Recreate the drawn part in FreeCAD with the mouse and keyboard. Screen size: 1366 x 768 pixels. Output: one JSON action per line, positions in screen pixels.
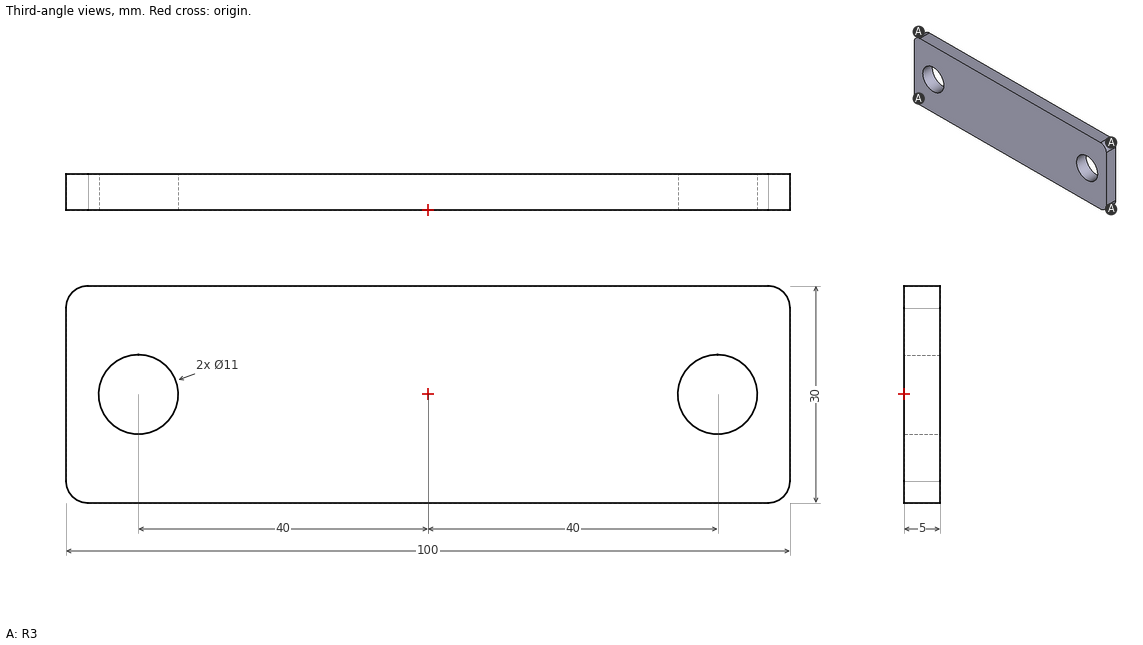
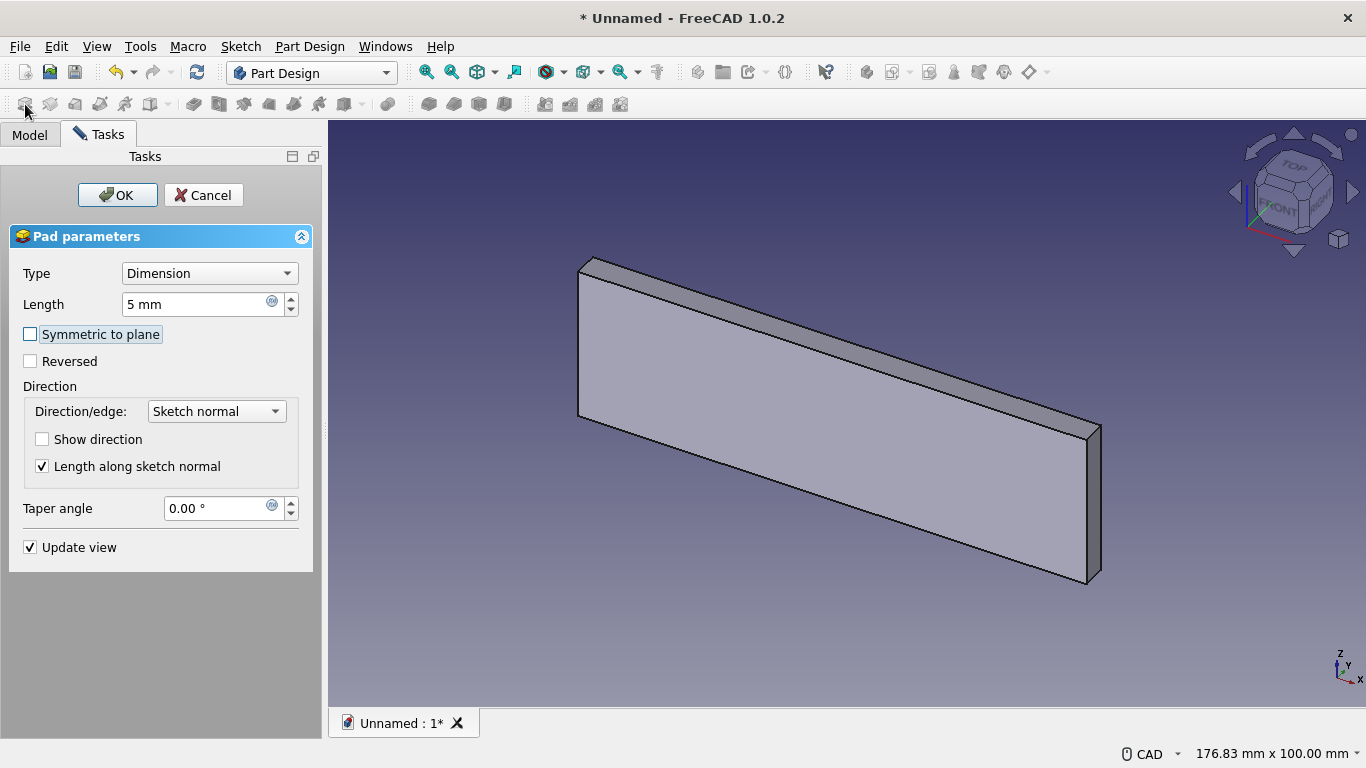
{"action": "left_click", "coordinate": [31, 361]}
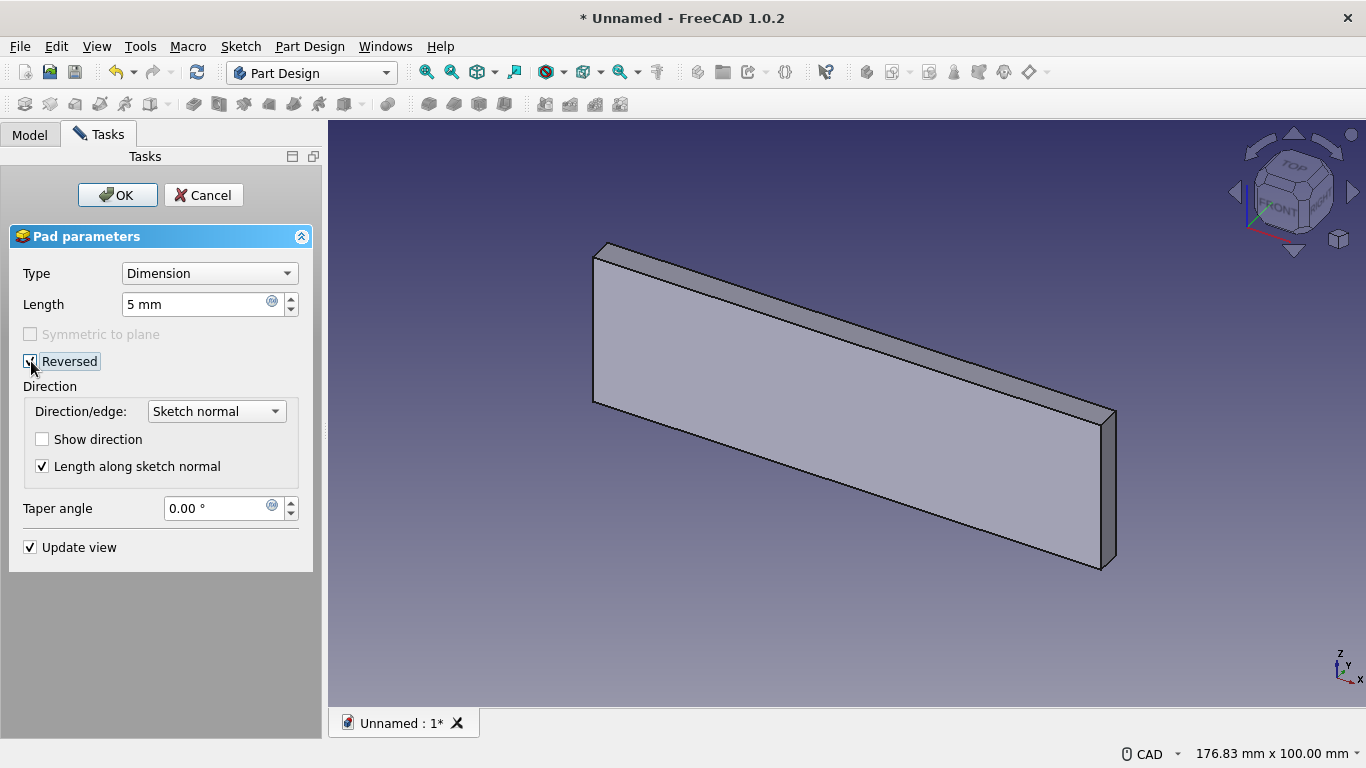
{"action": "left_click", "coordinate": [118, 195]}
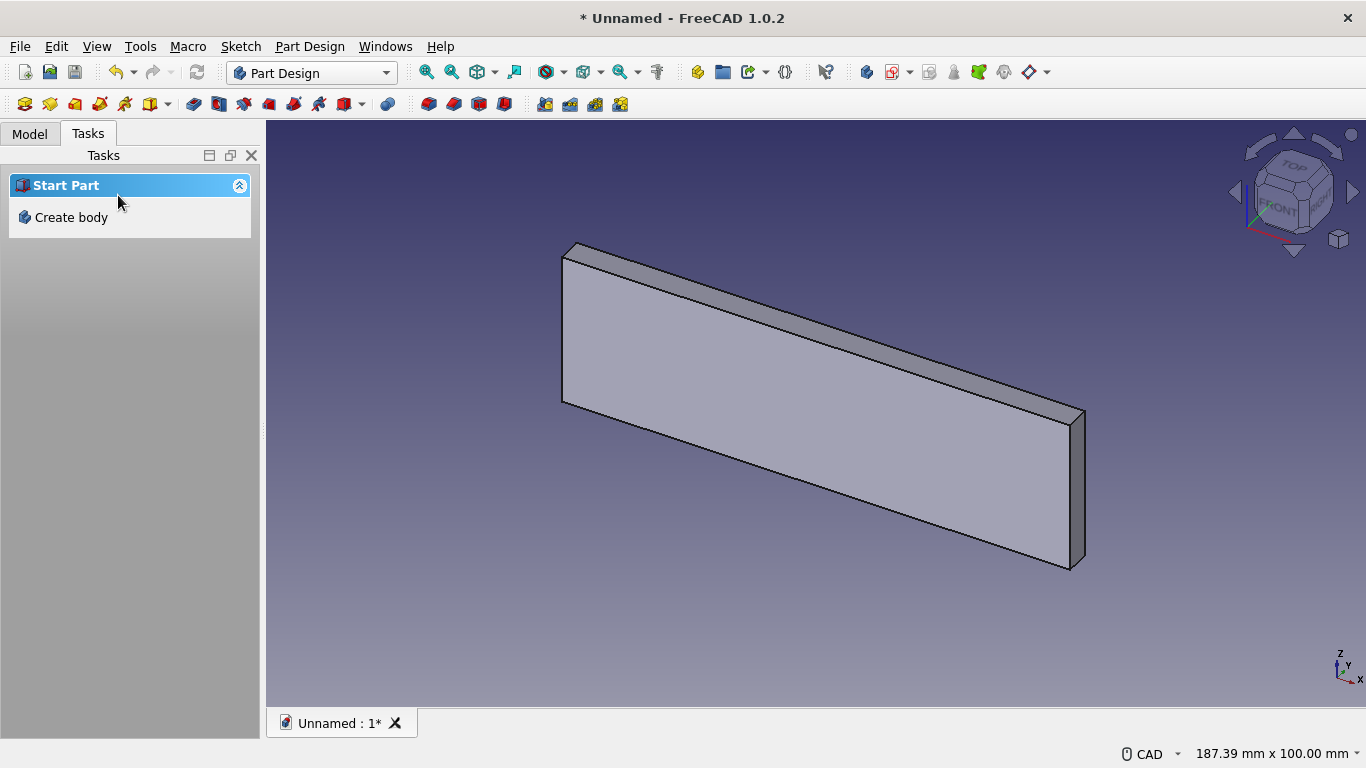
{"action": "left_click", "coordinate": [1078, 417]}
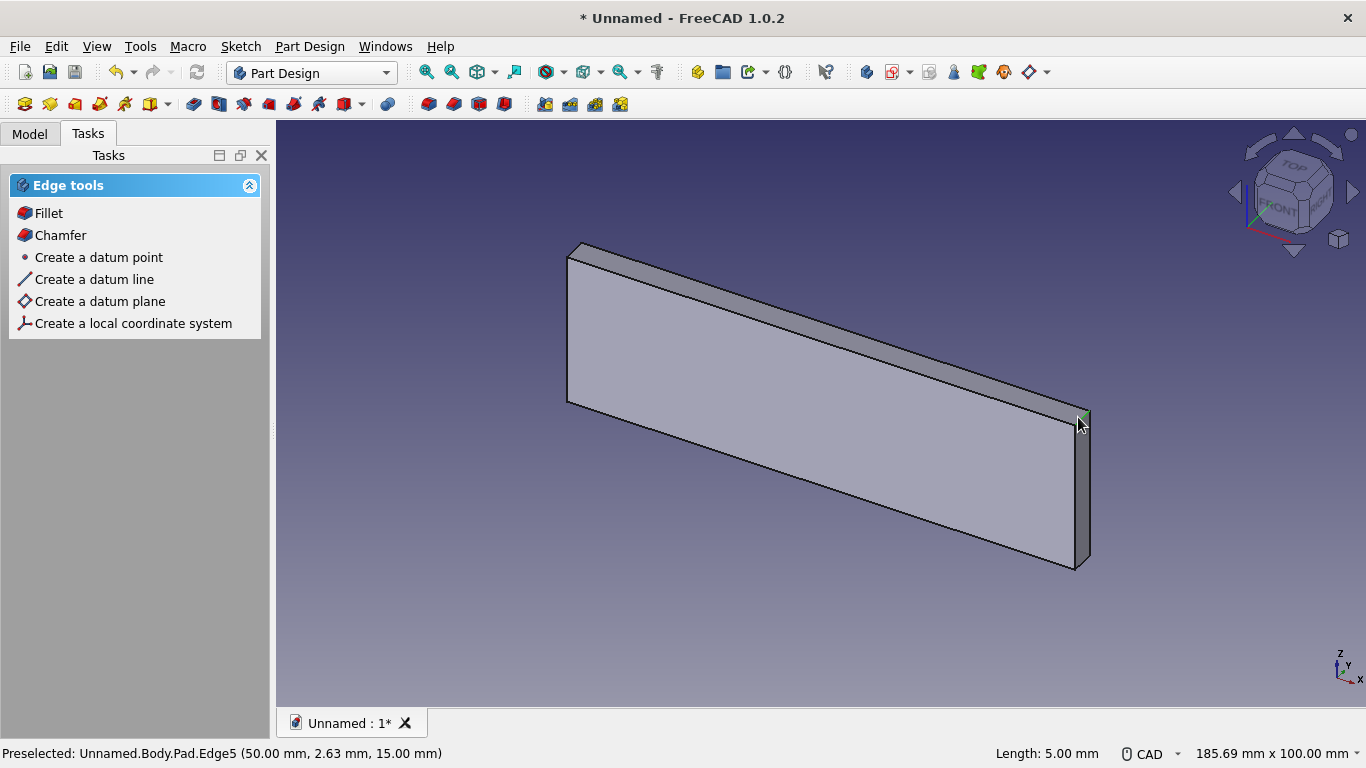
{"action": "key", "text": "0"}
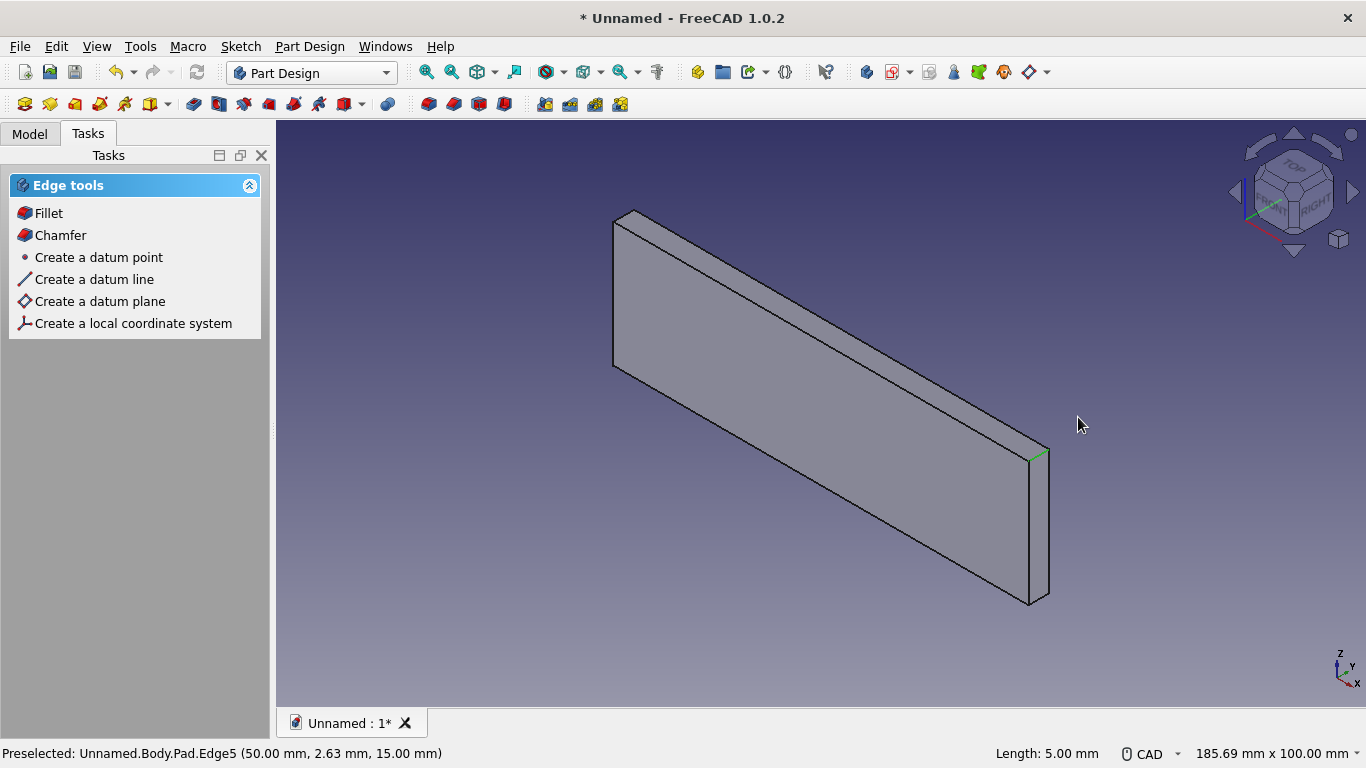
{"action": "key", "text": "2"}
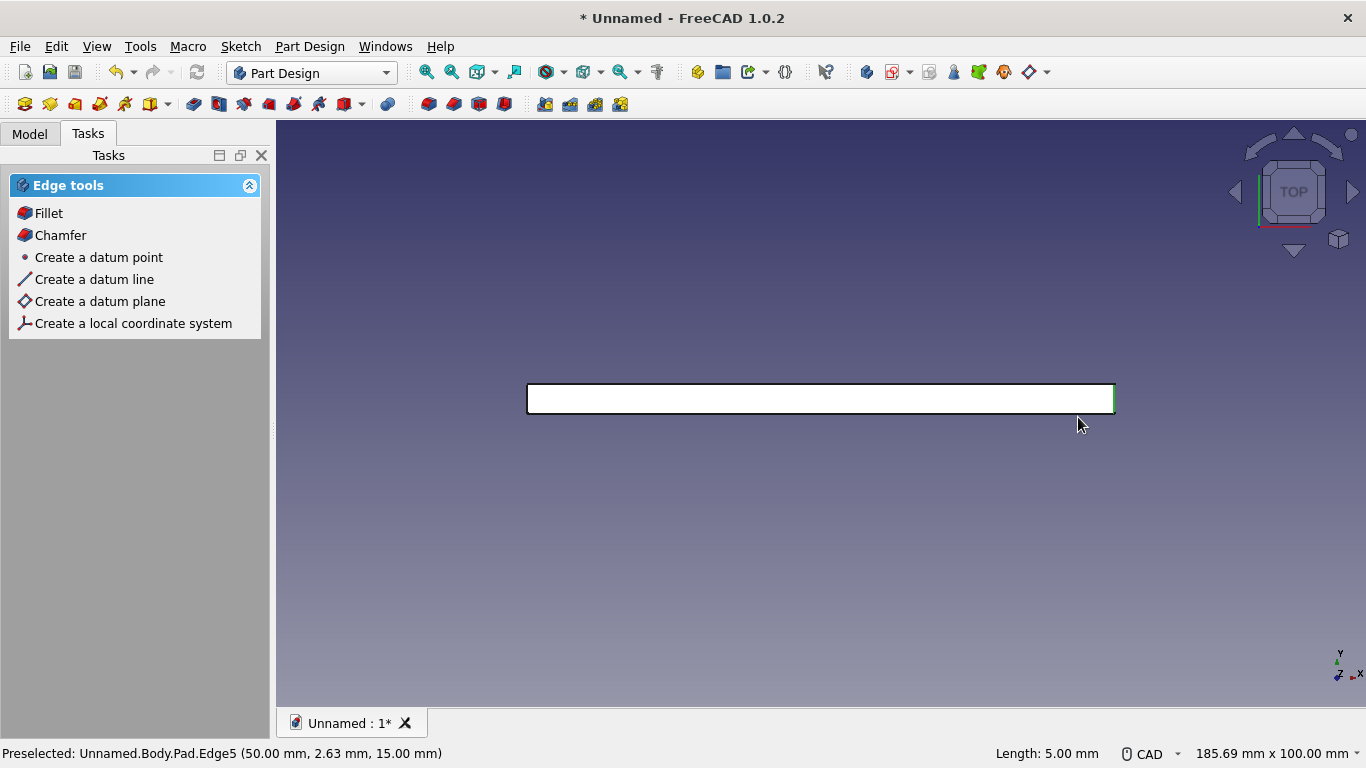
{"action": "left_click", "coordinate": [527, 398], "text": "ctrl"}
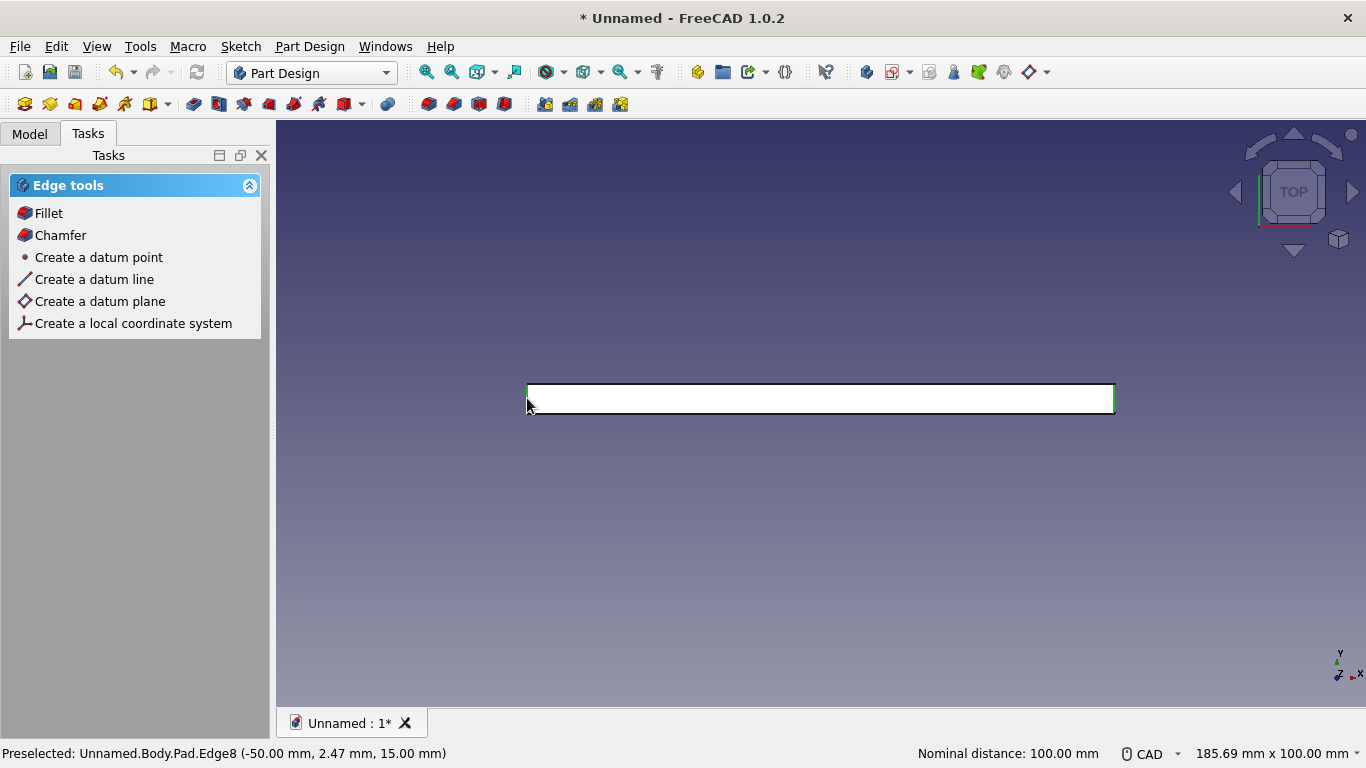
{"action": "key", "text": "1"}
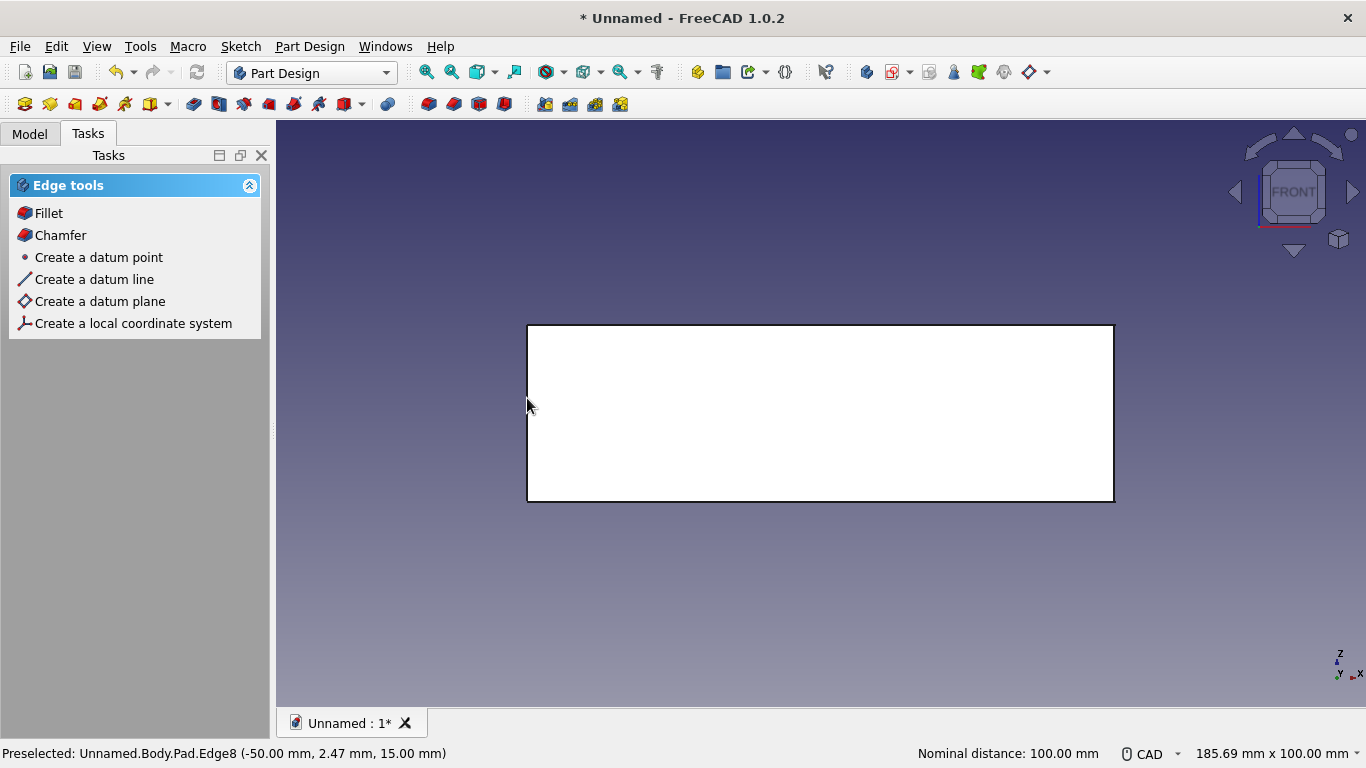
{"action": "key", "text": "3"}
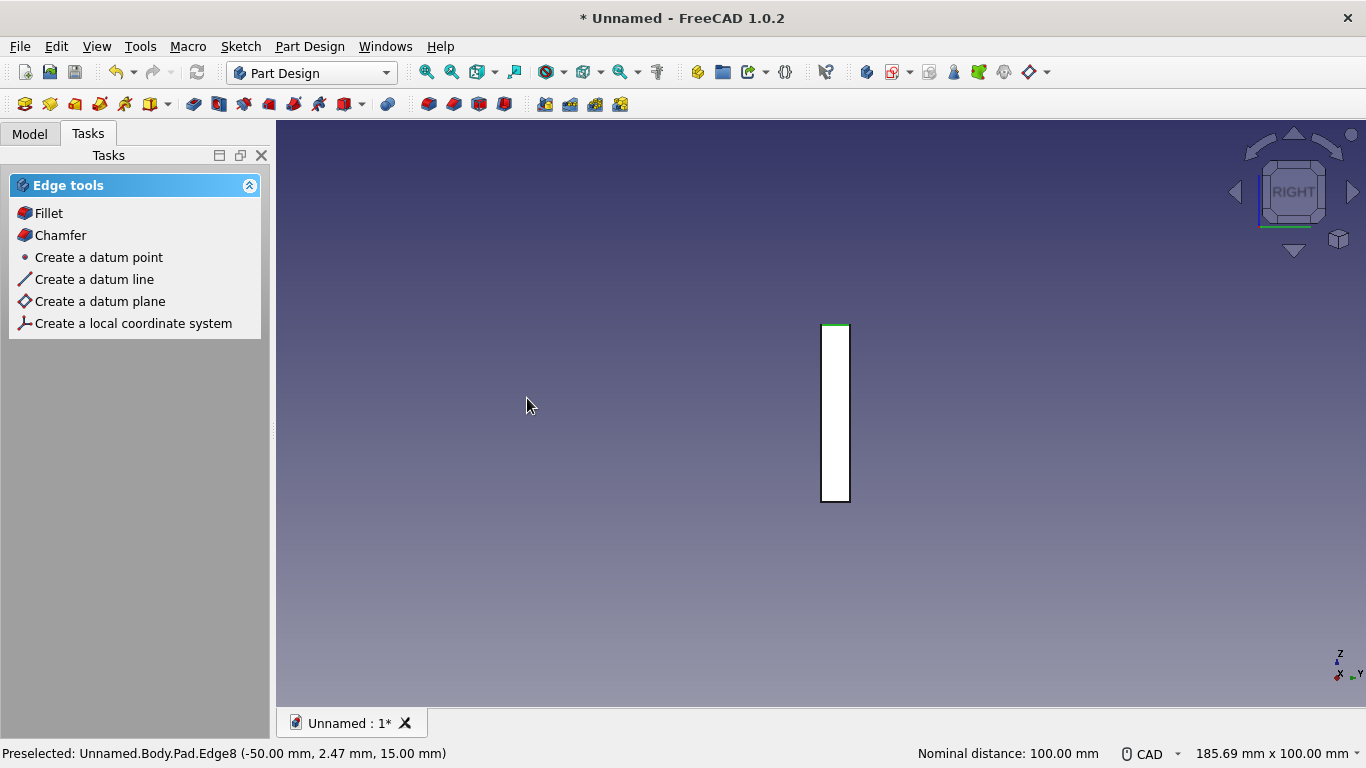
{"action": "left_click", "coordinate": [427, 72]}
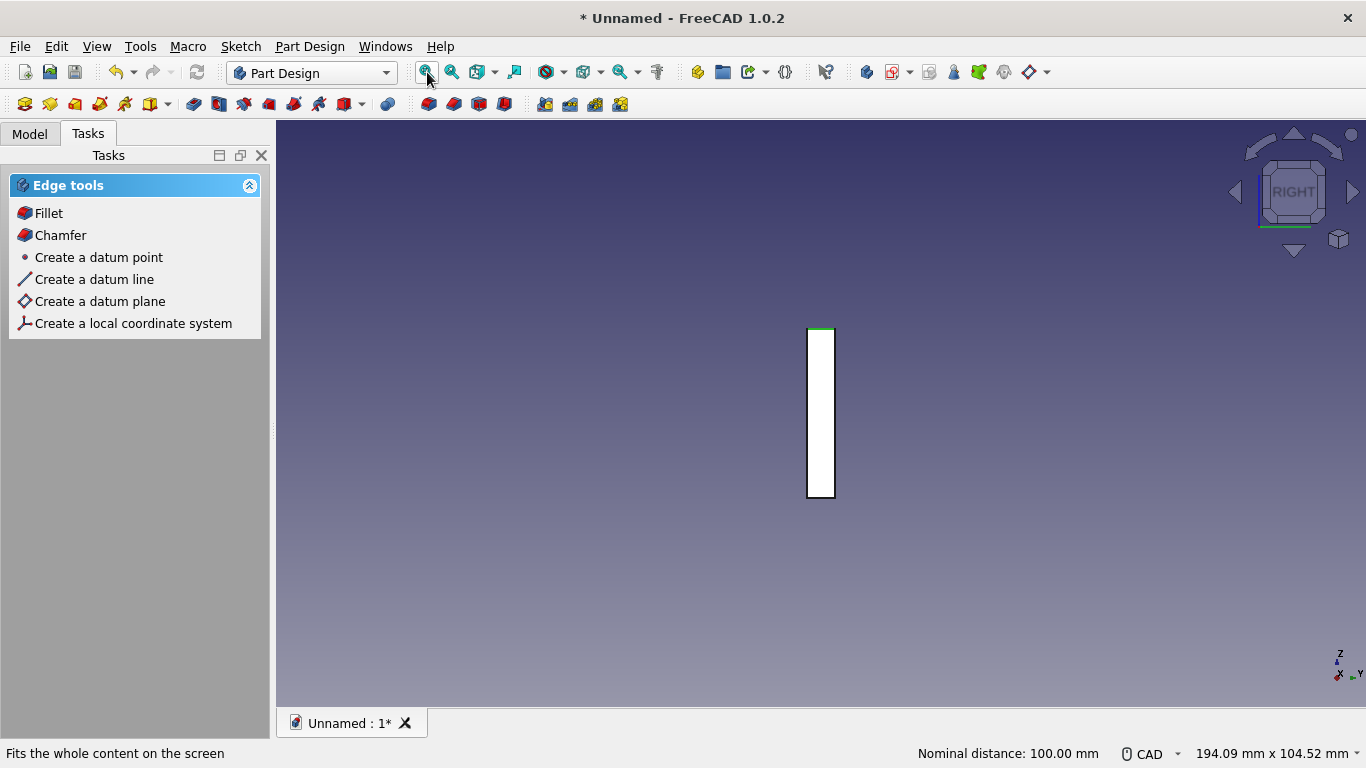
{"action": "left_click", "coordinate": [821, 497], "text": "ctrl"}